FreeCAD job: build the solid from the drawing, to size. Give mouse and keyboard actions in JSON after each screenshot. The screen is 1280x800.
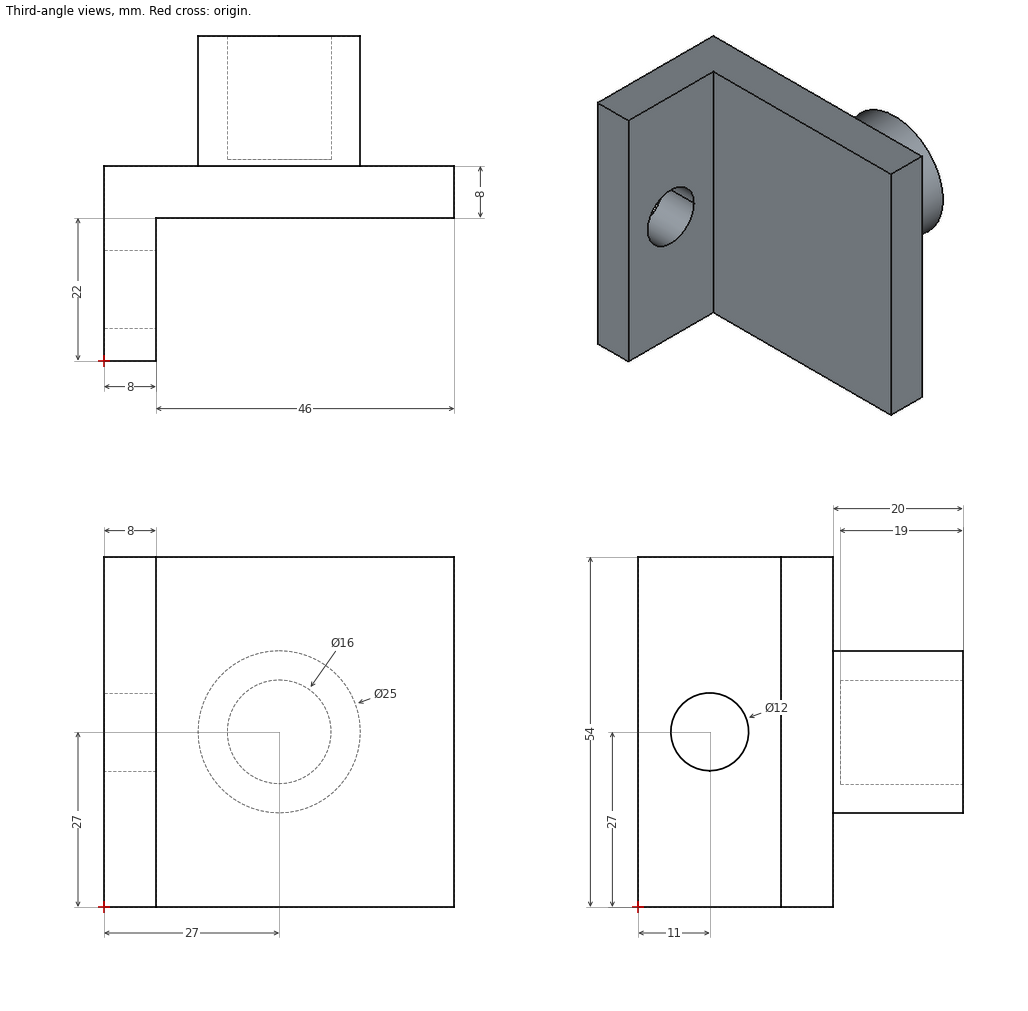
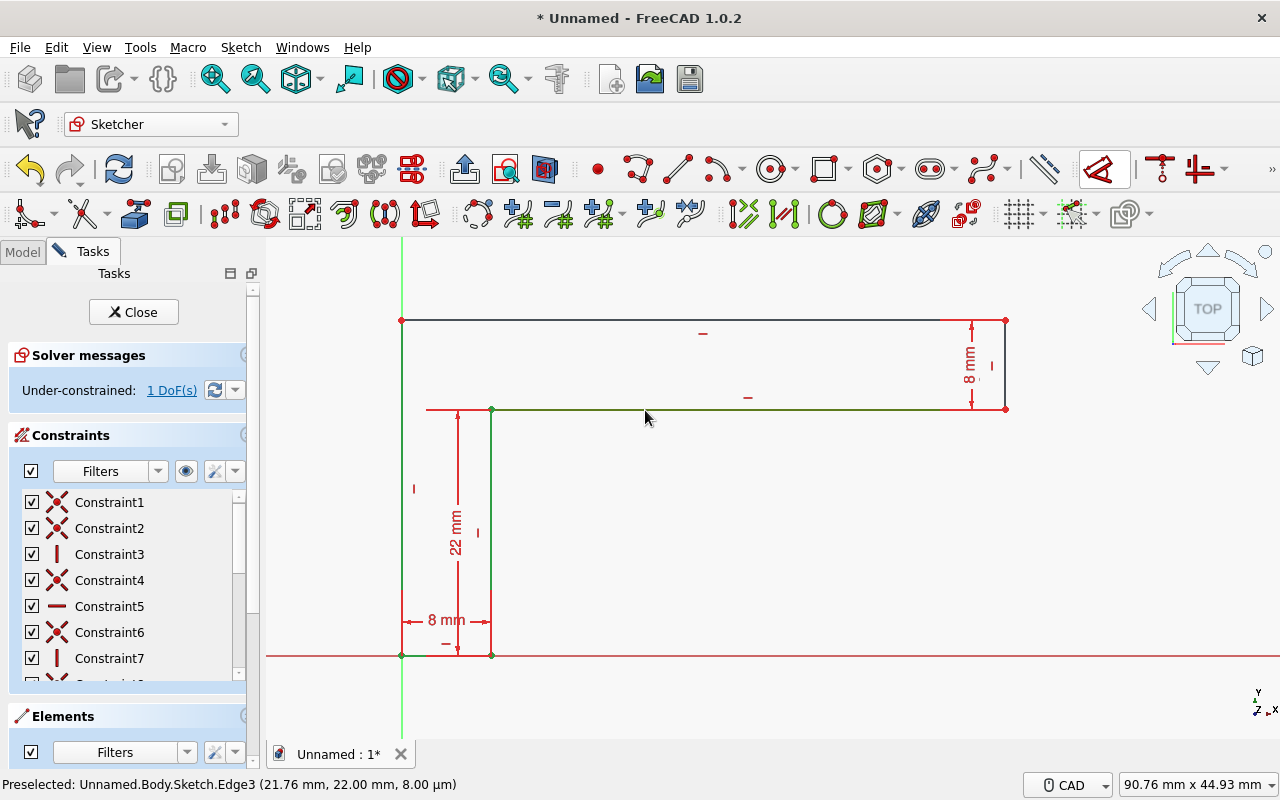
{"action": "key", "text": "l"}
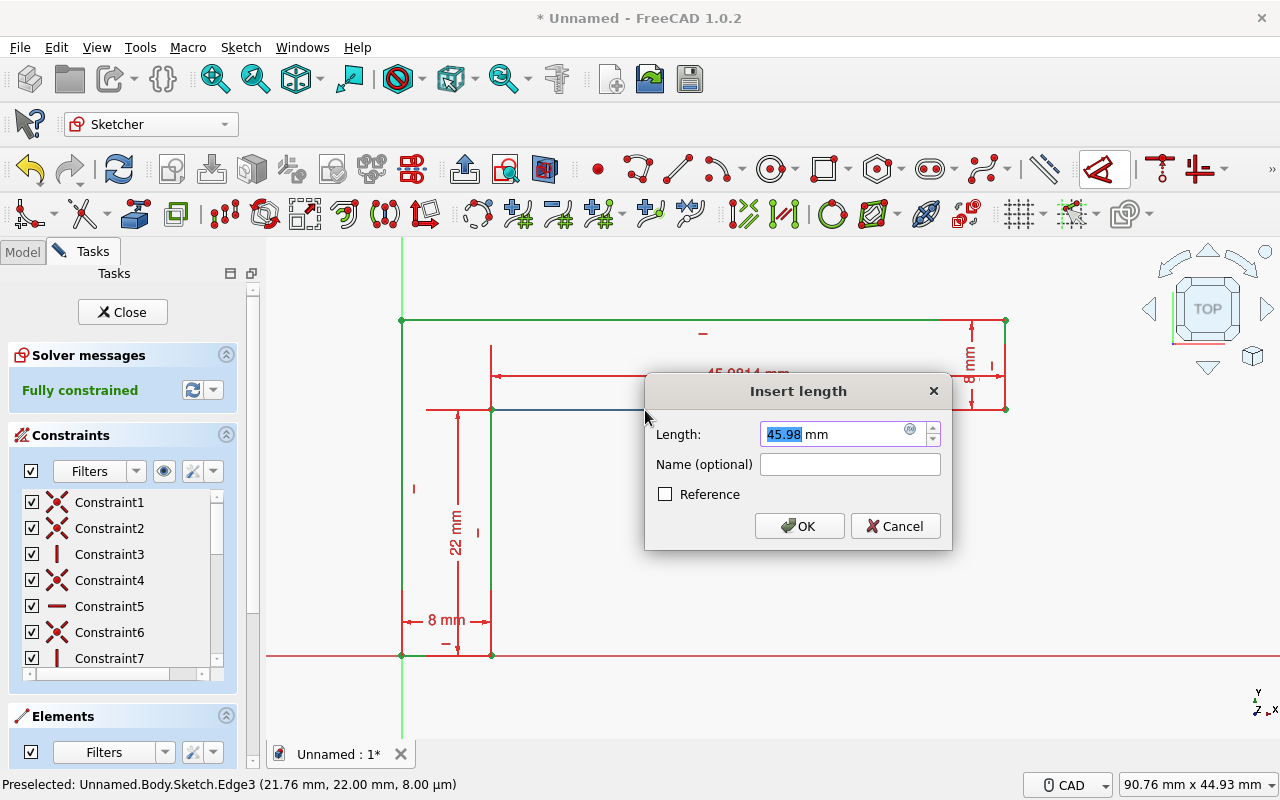
{"action": "type", "text": "46"}
{"action": "key", "text": "Return"}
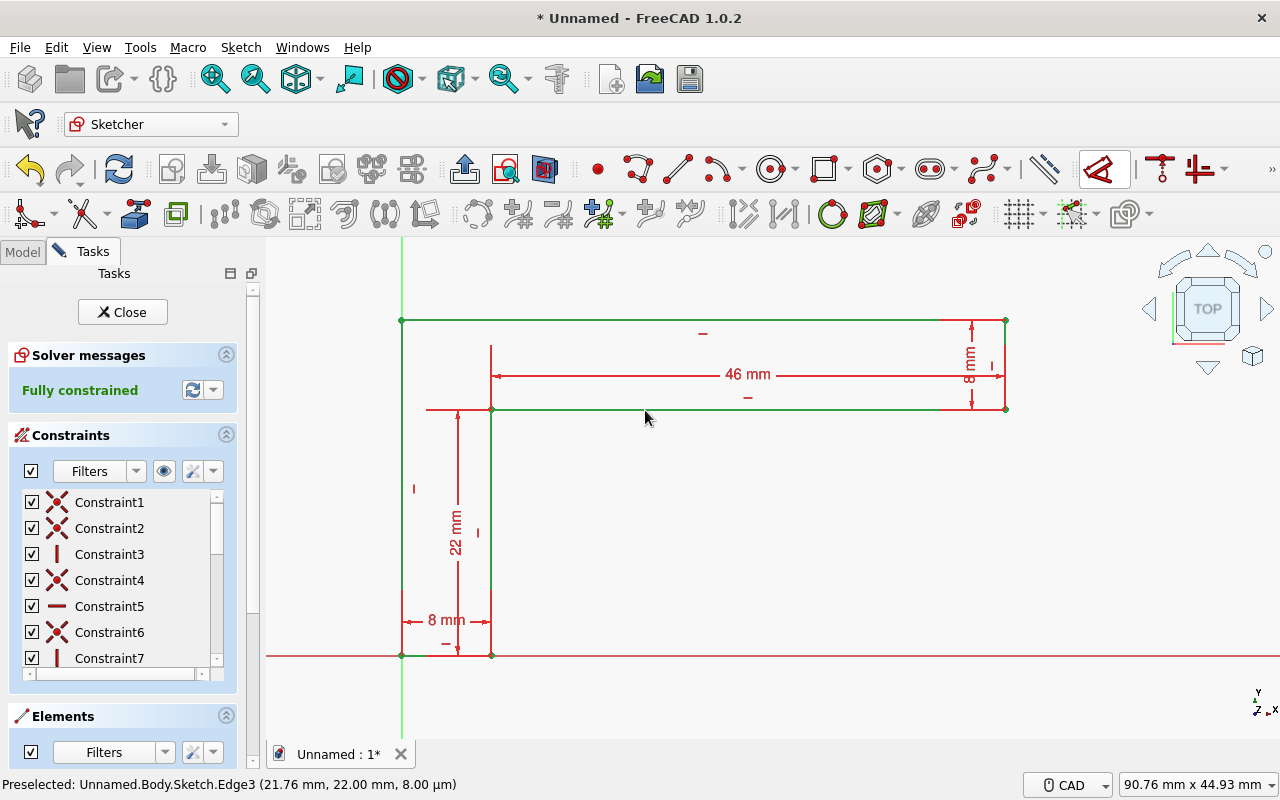
{"action": "left_click", "coordinate": [123, 312]}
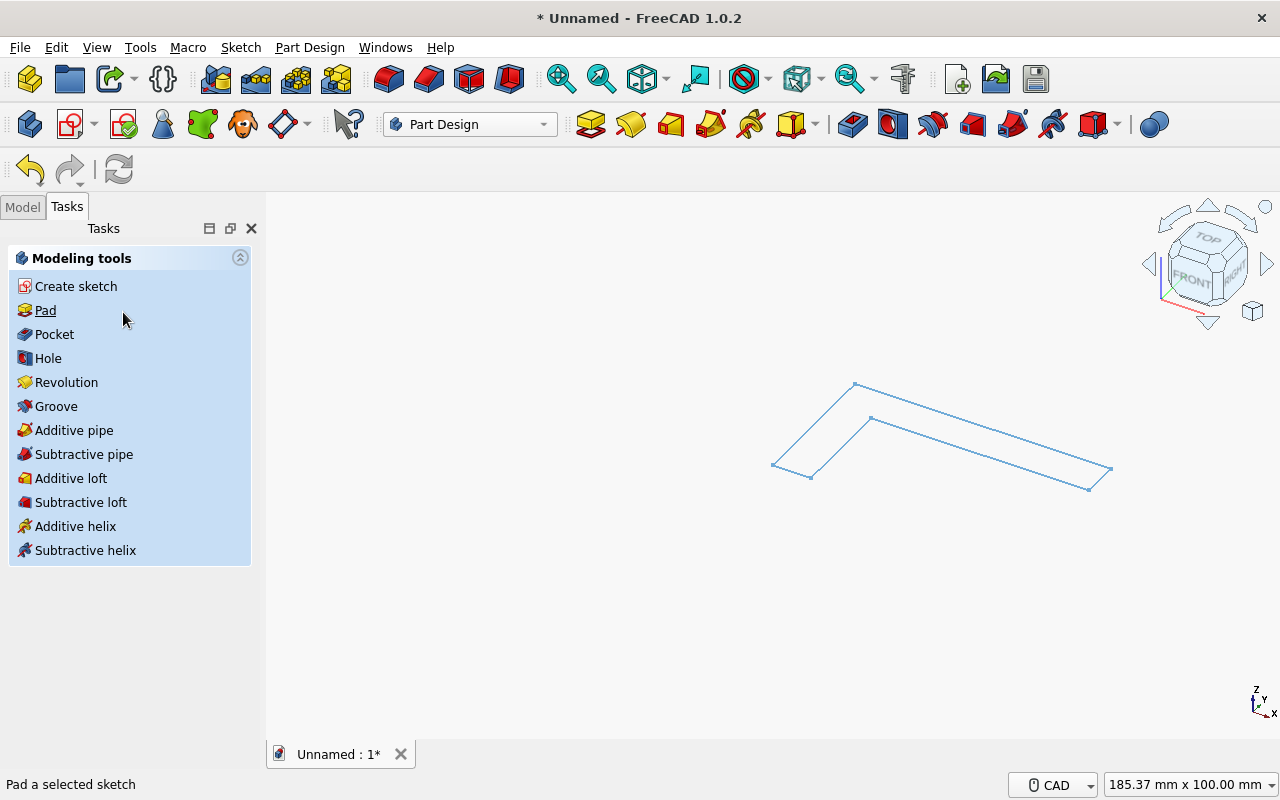
{"action": "left_click", "coordinate": [592, 124]}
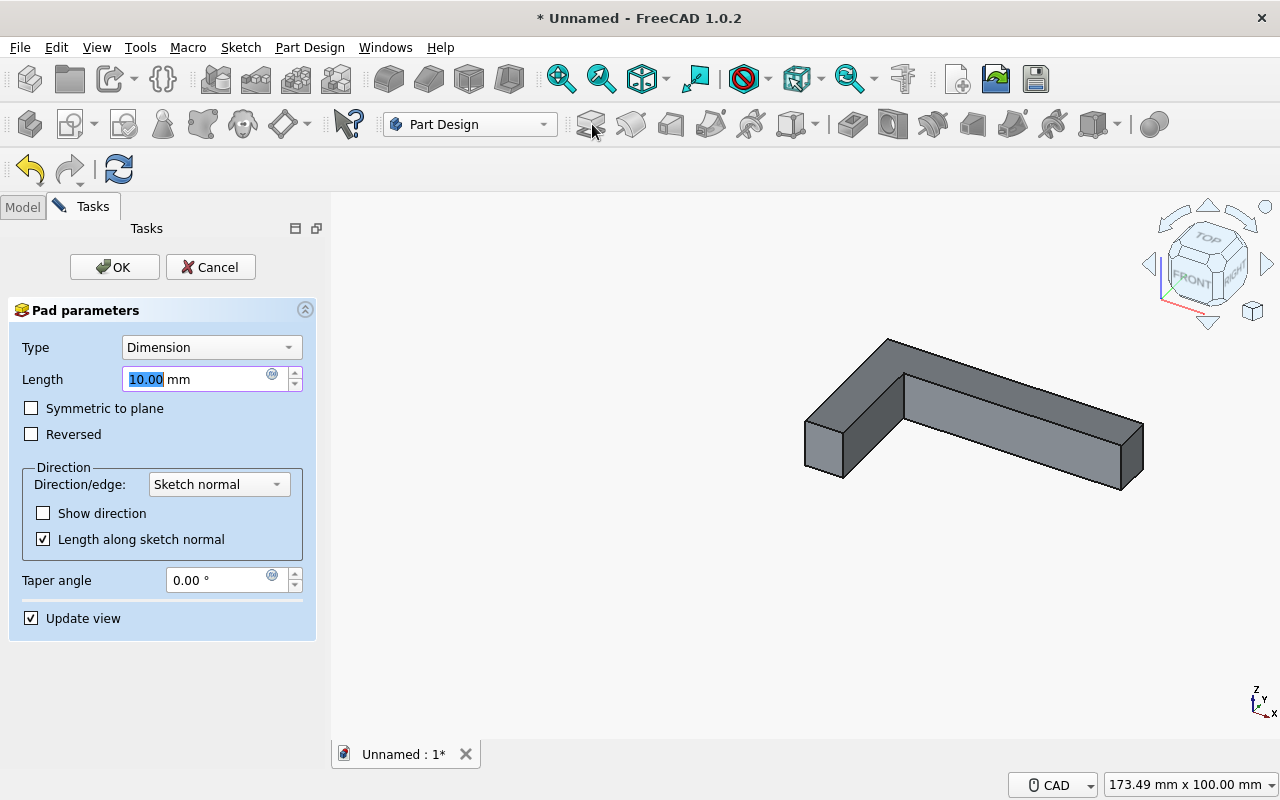
{"action": "type", "text": "54"}
{"action": "key", "text": "Tab"}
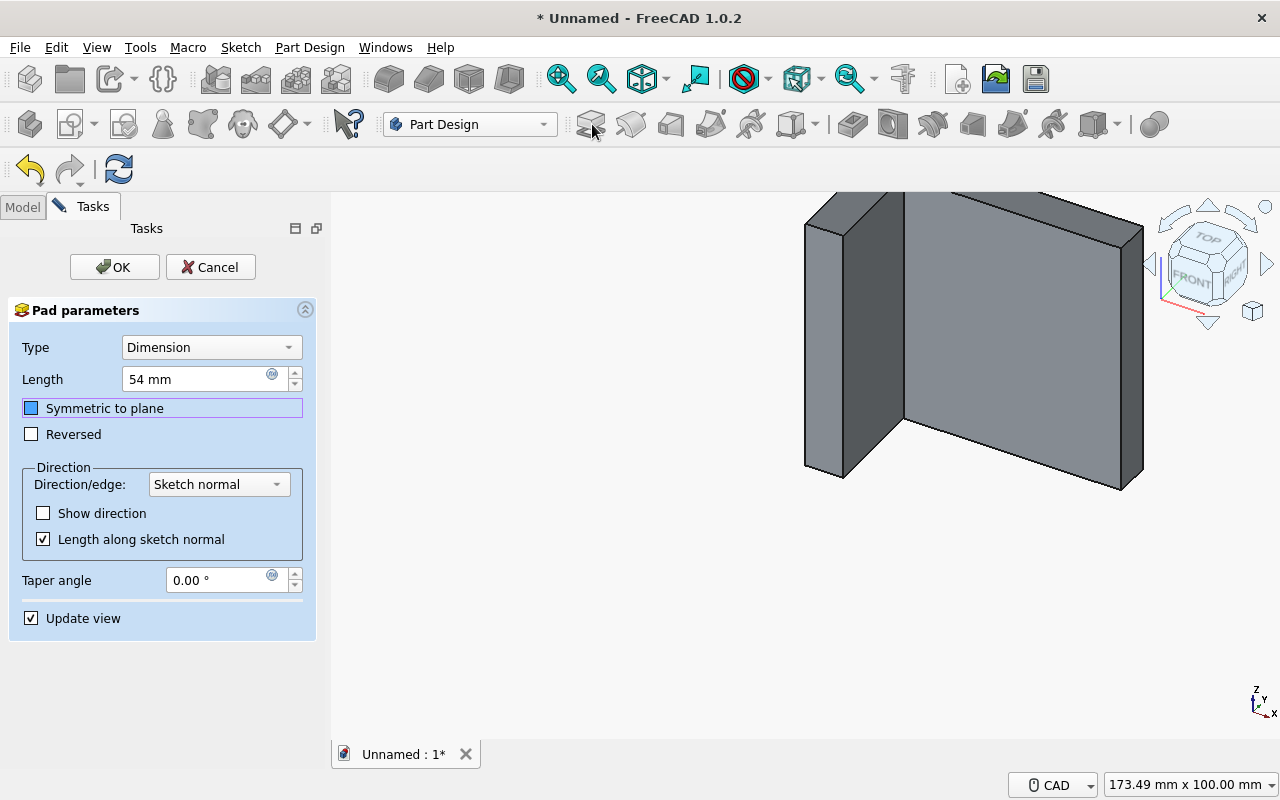
{"action": "left_click", "coordinate": [115, 267]}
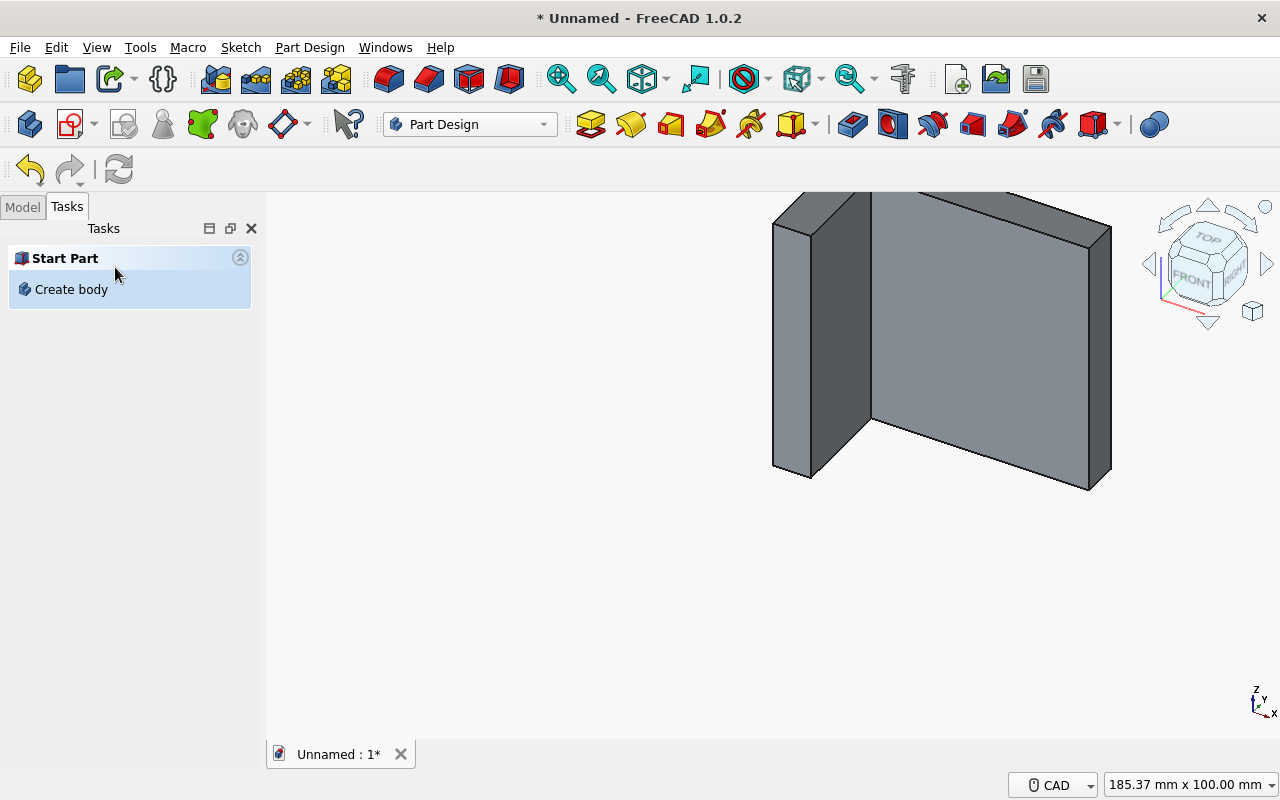
{"action": "left_click", "coordinate": [562, 80]}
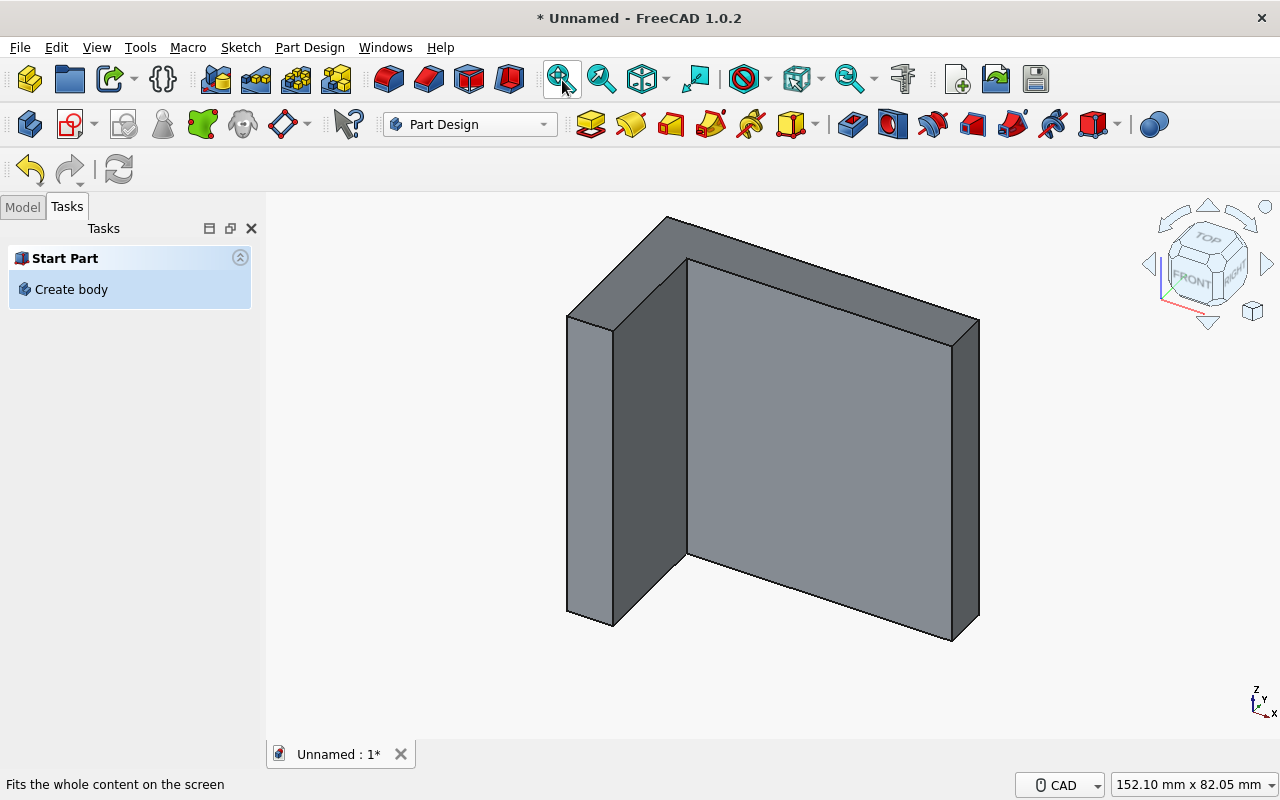
{"action": "key", "text": "4"}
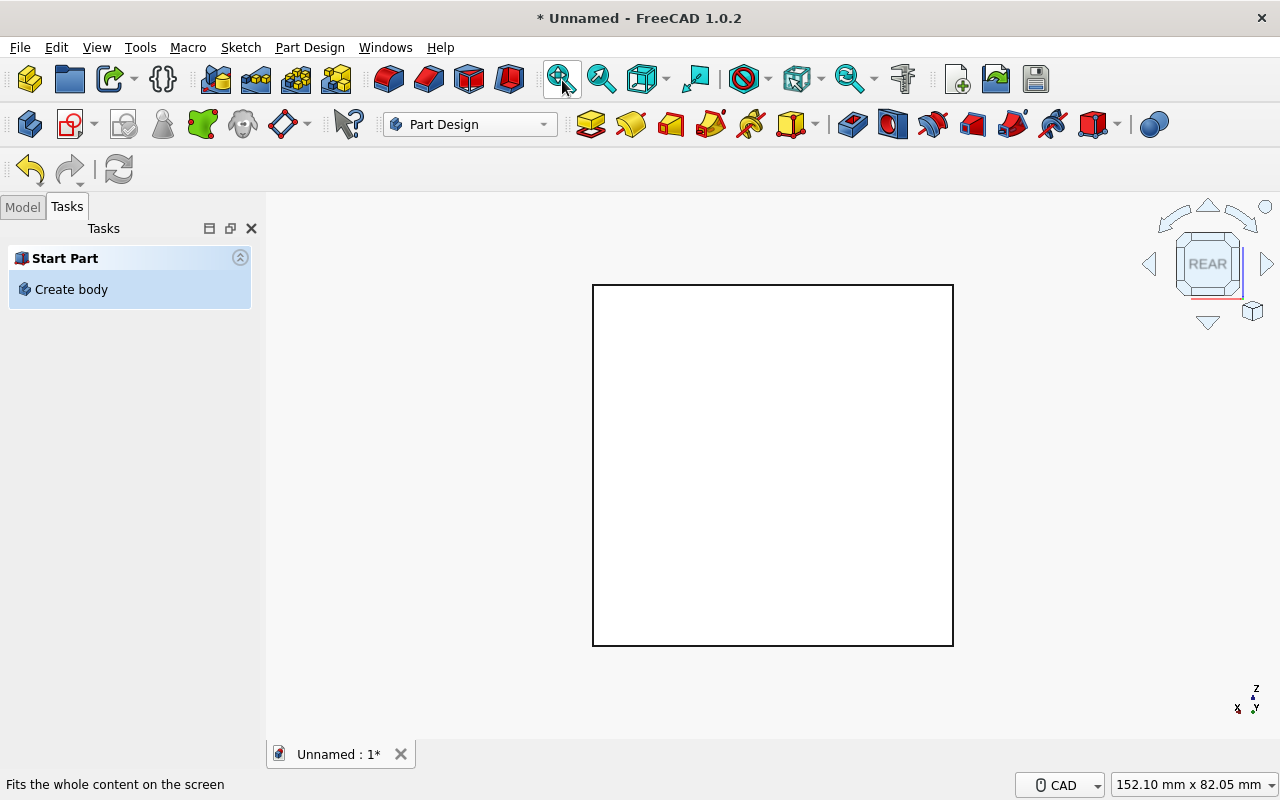
{"action": "left_click", "coordinate": [773, 465]}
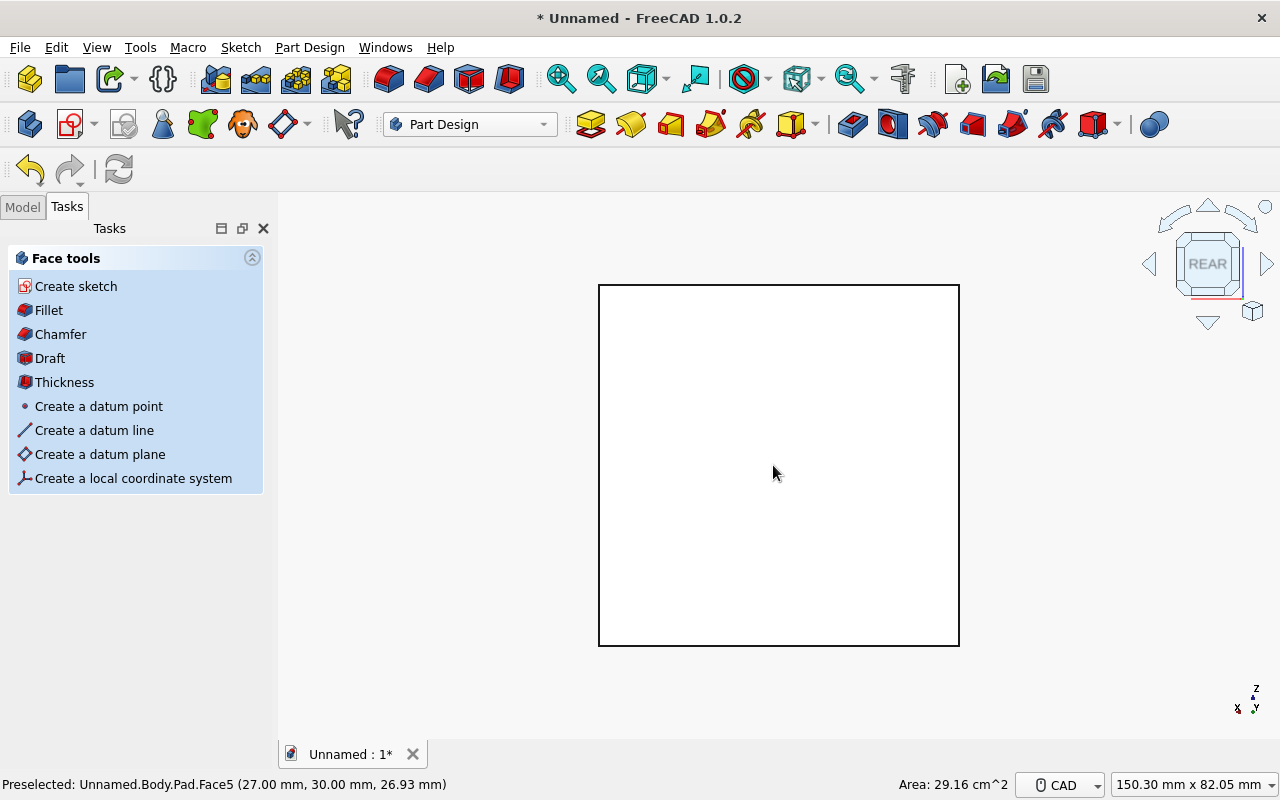
{"action": "left_click", "coordinate": [70, 124]}